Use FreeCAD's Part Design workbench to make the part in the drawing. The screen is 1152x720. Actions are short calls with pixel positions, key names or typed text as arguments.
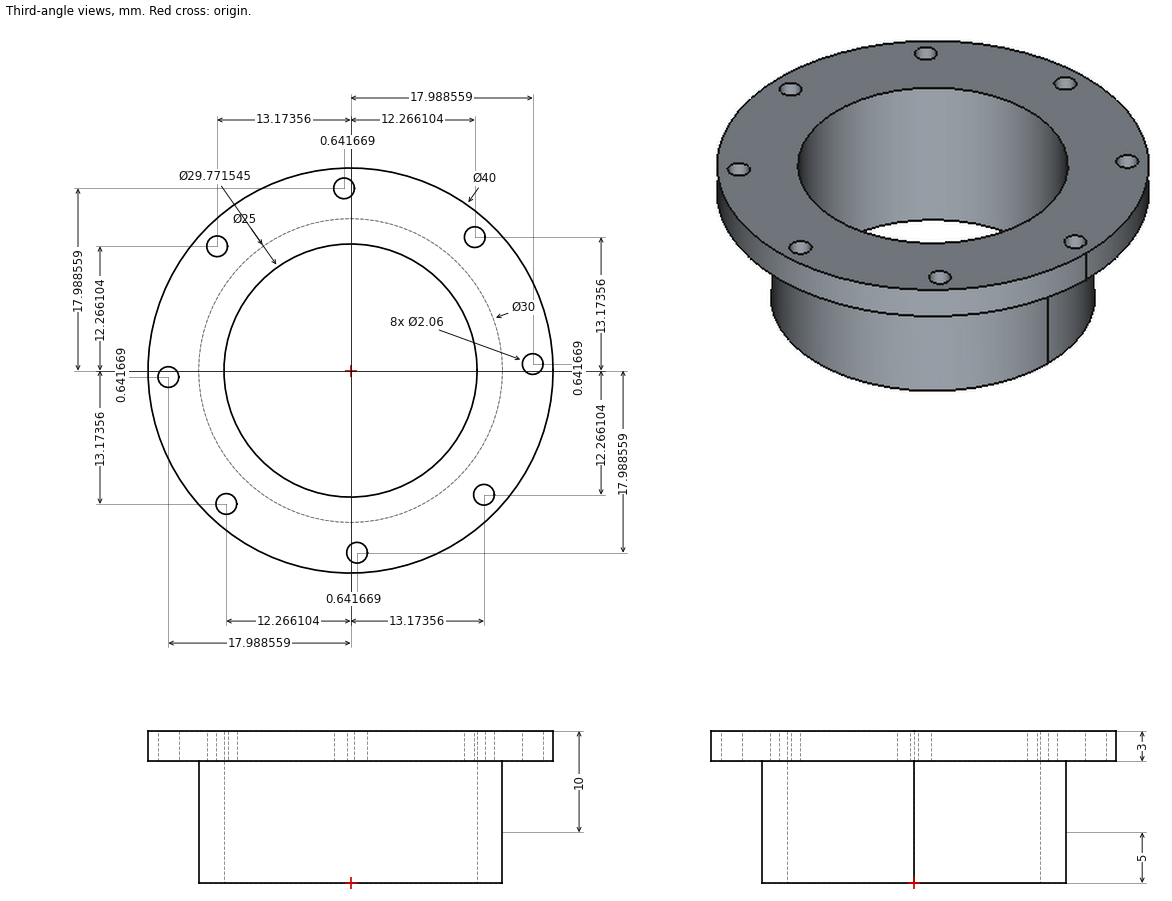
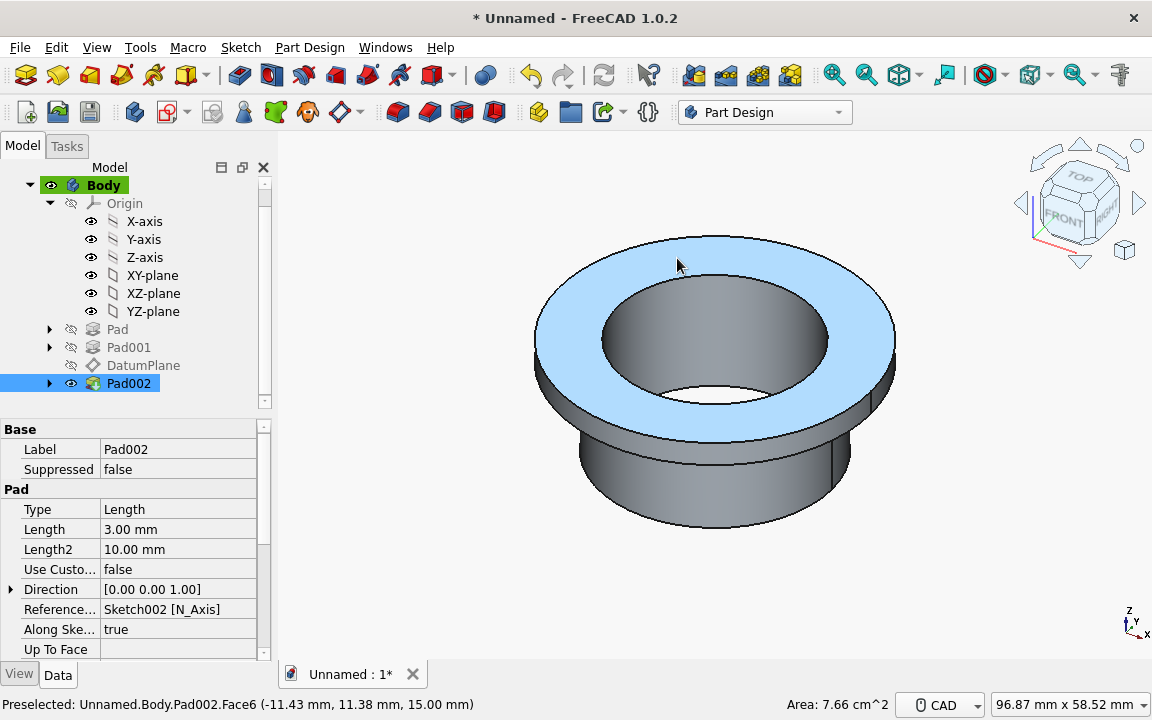
click(168, 112)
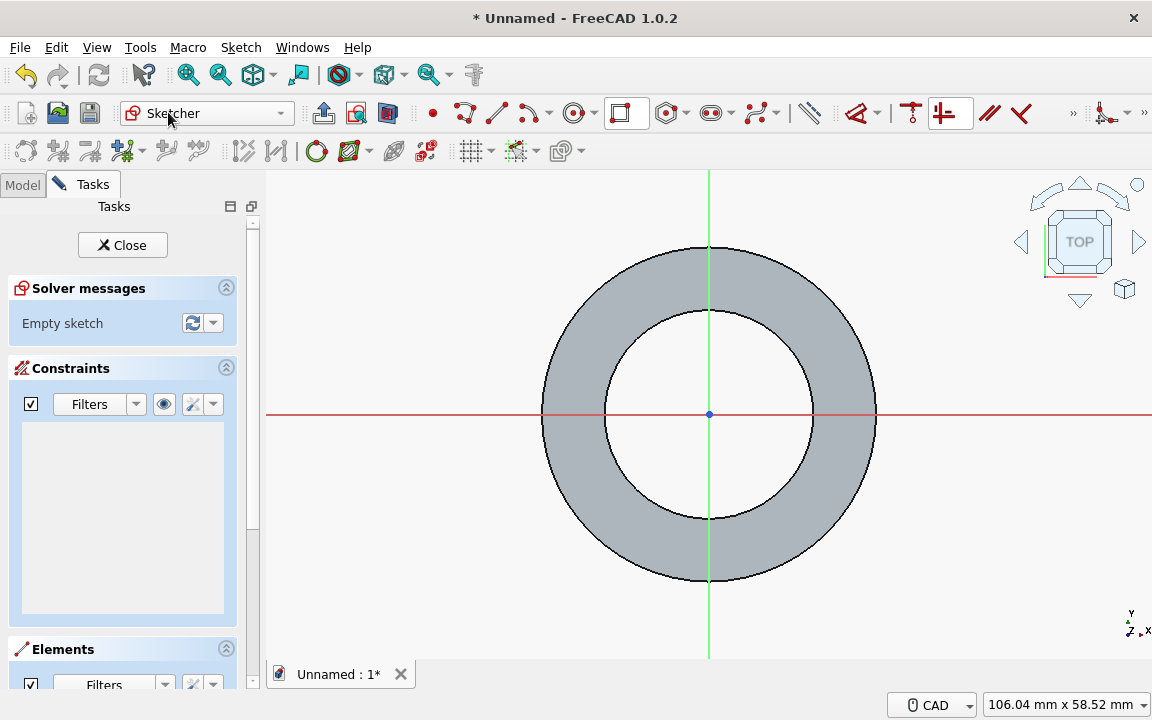
key(g)
key(c)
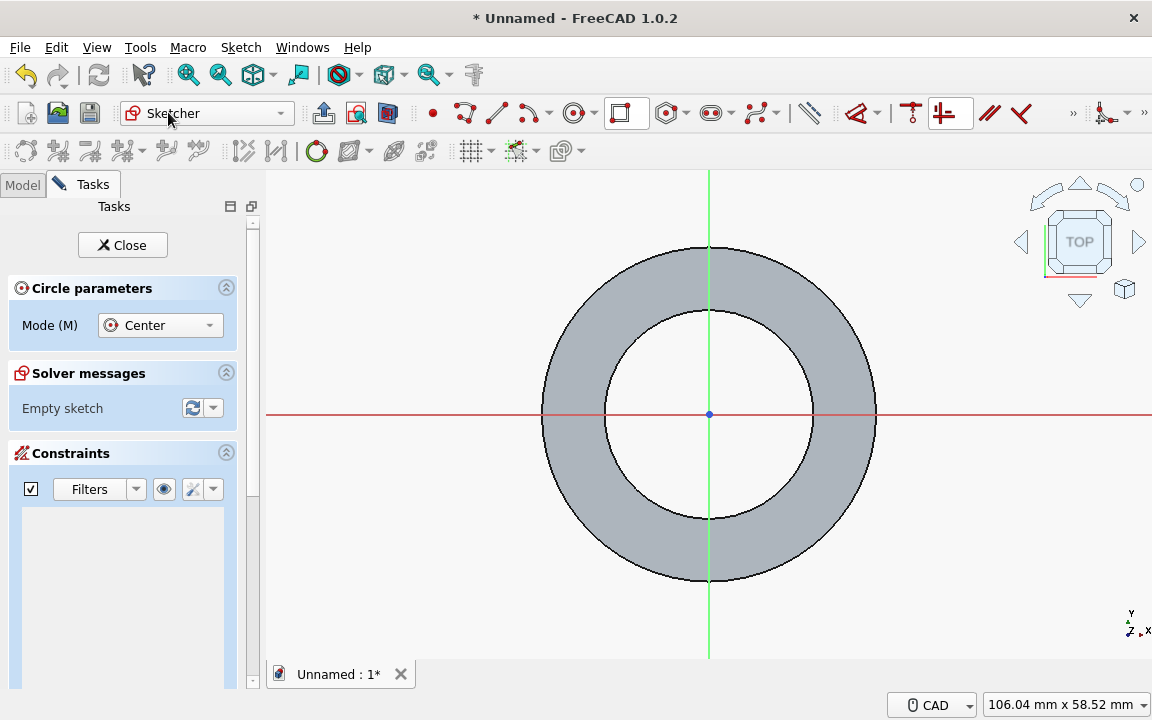
scroll(859, 409, up, 6)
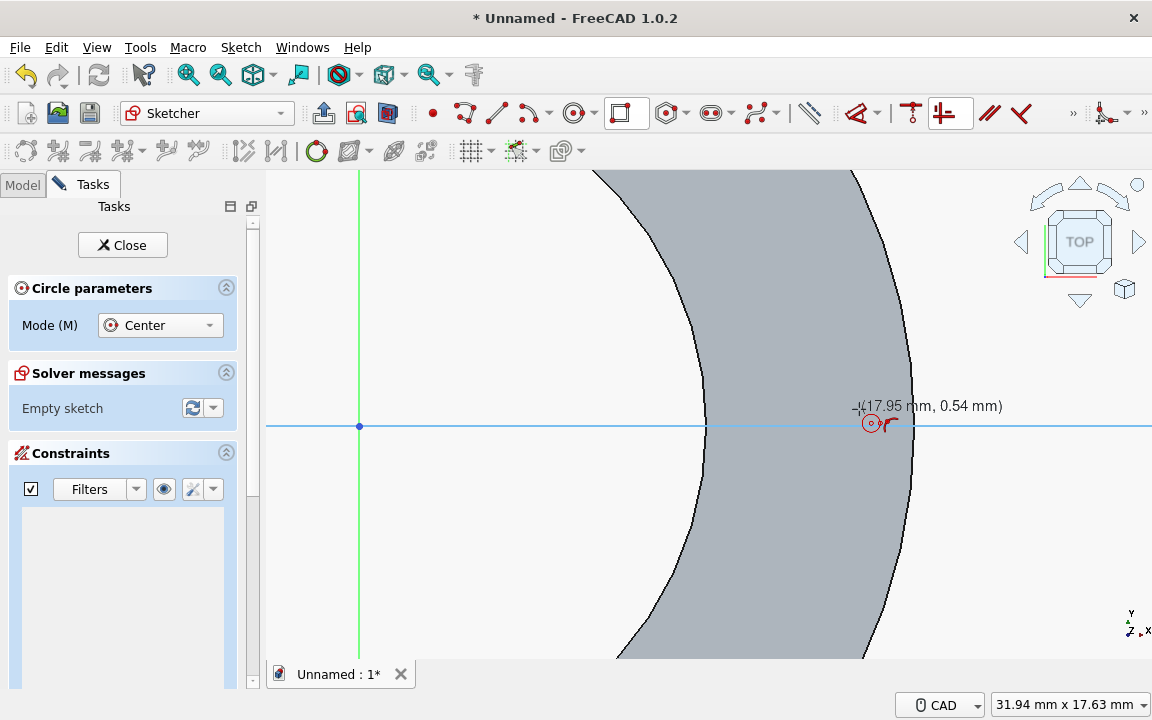
click(858, 408)
click(879, 388)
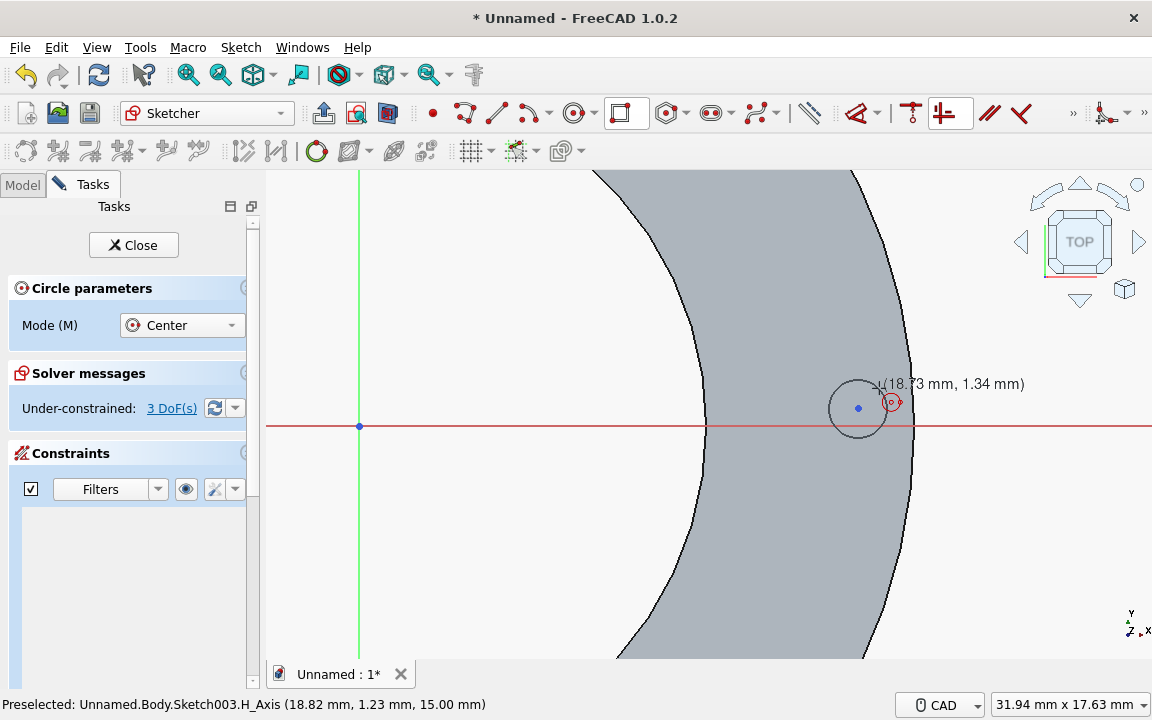
scroll(762, 409, down, 6)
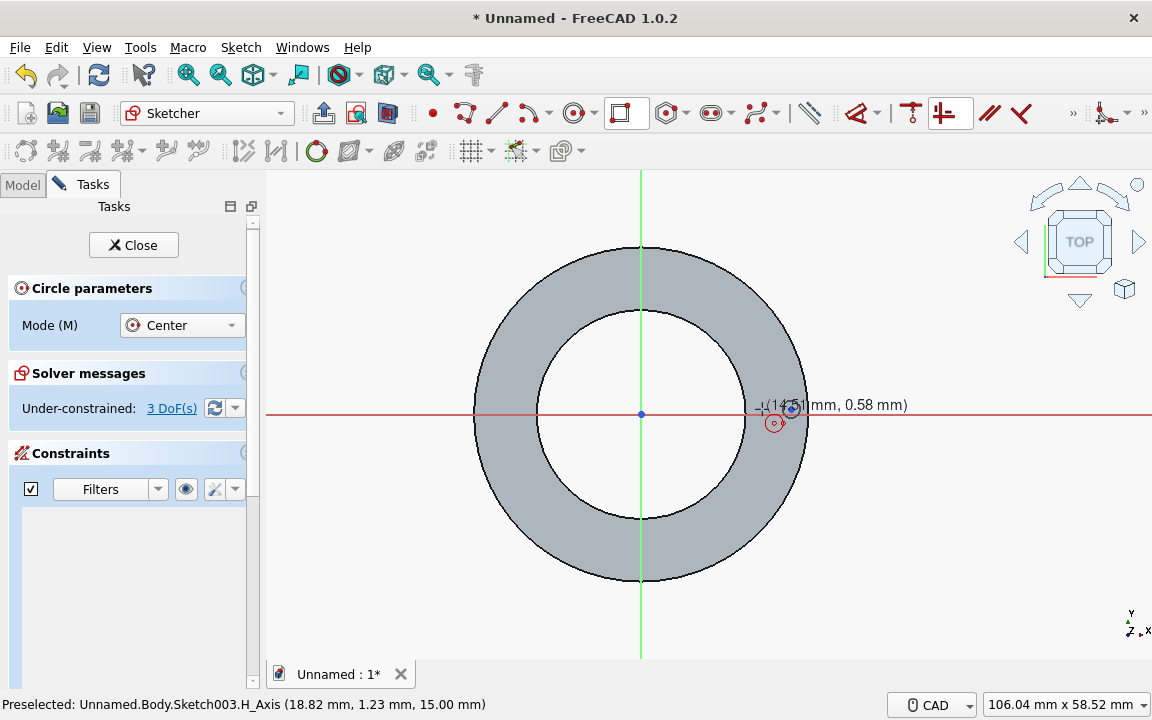
scroll(751, 517, up, 5)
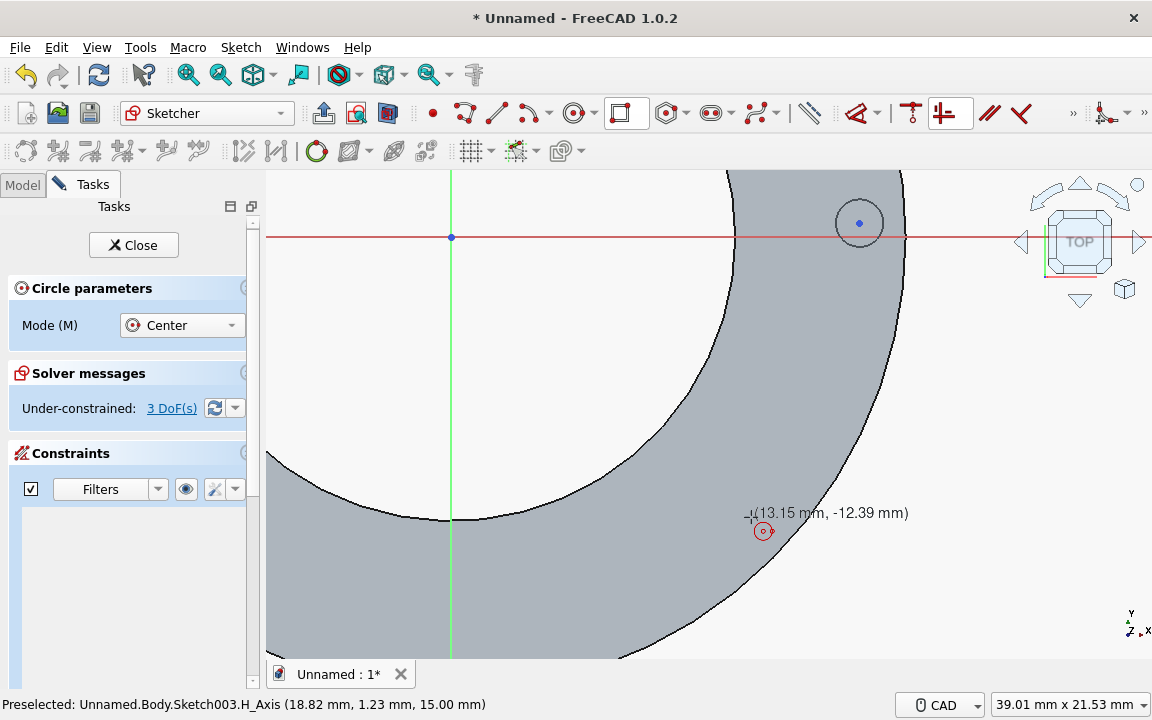
click(751, 516)
click(767, 499)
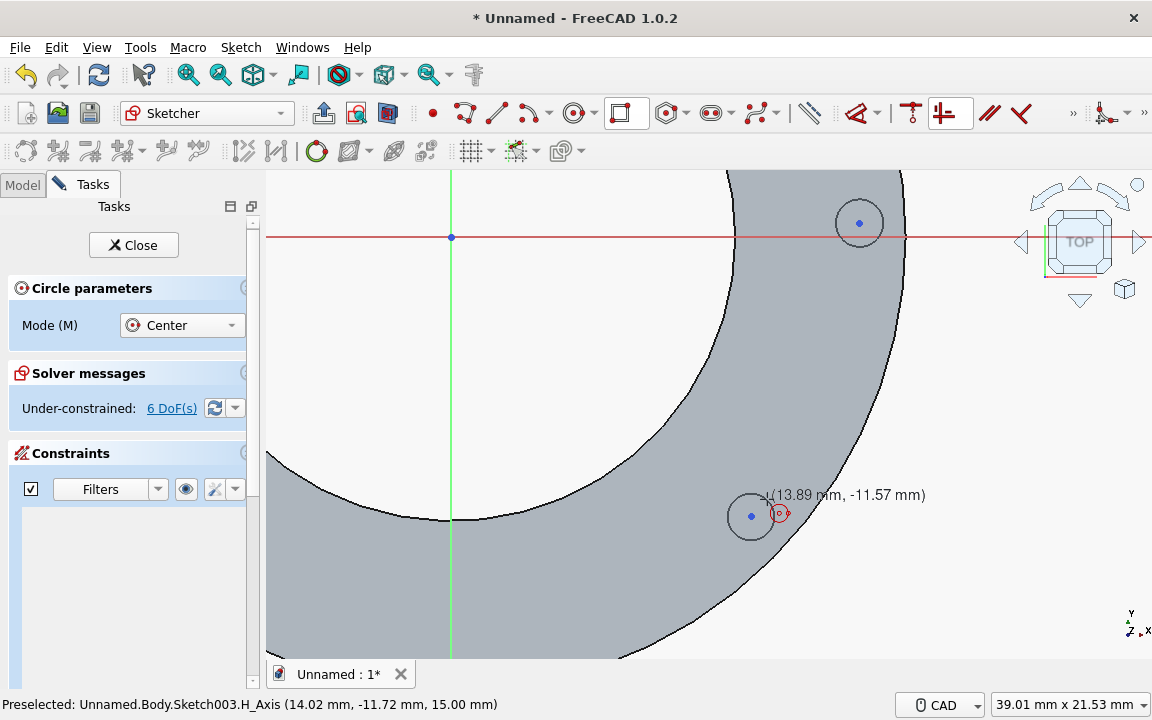
scroll(751, 518, down, 5)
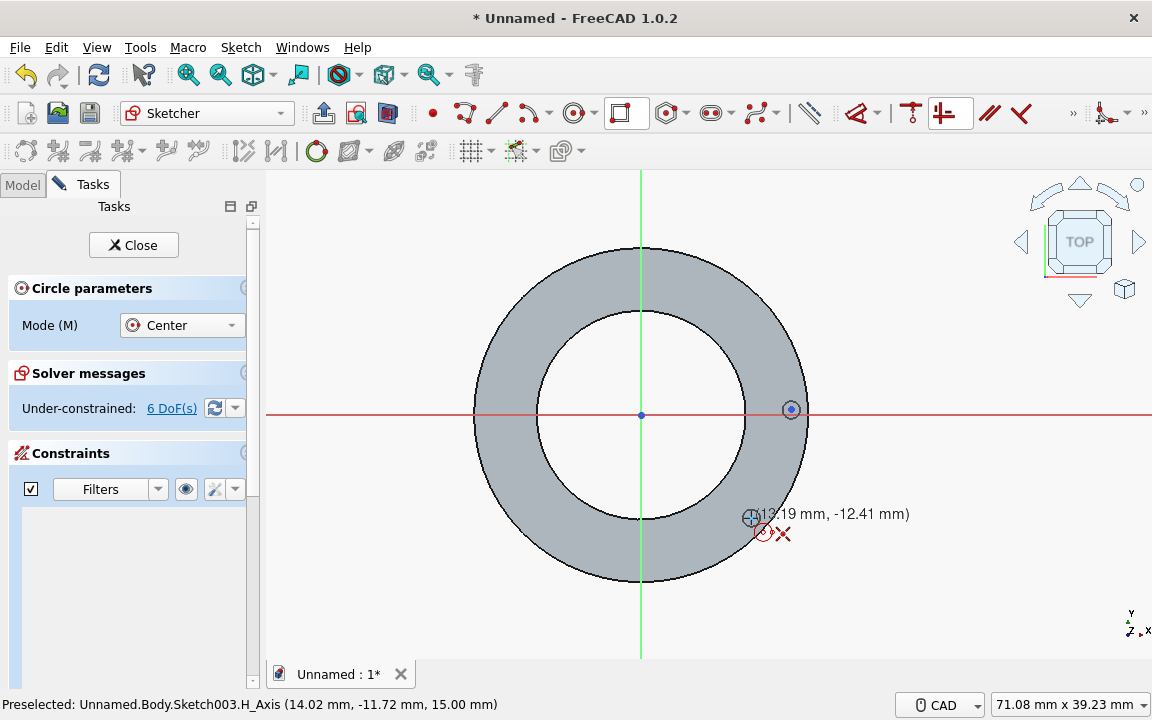
scroll(647, 565, up, 6)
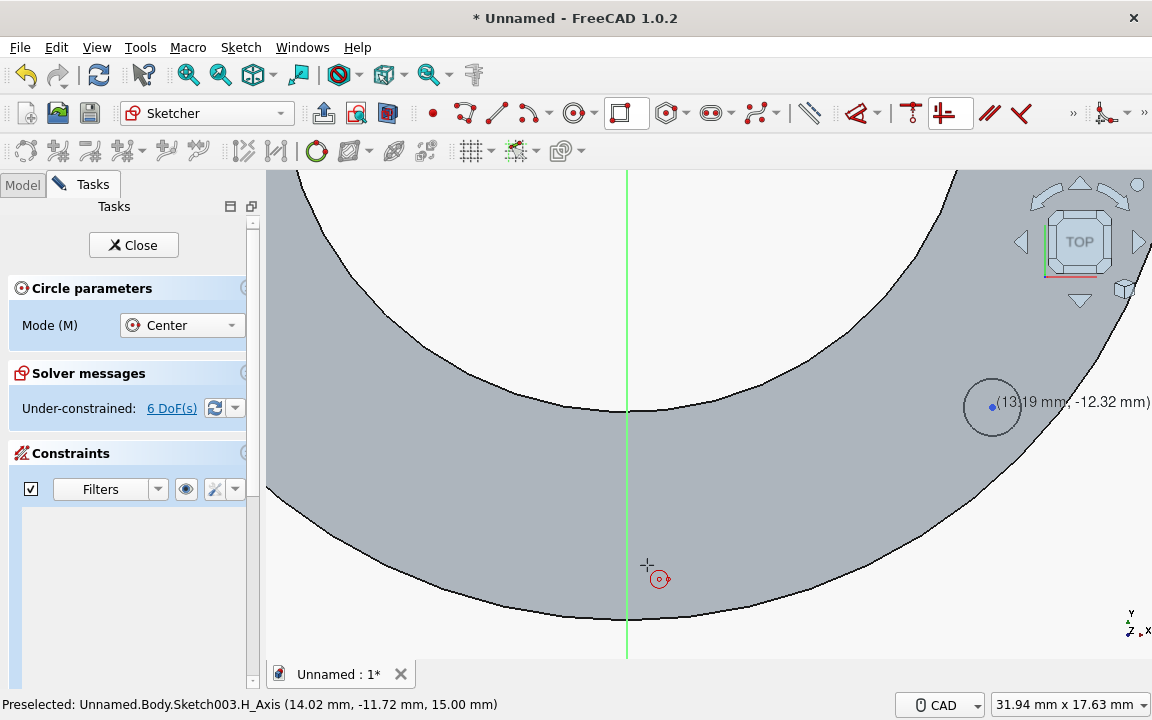
click(644, 565)
click(665, 544)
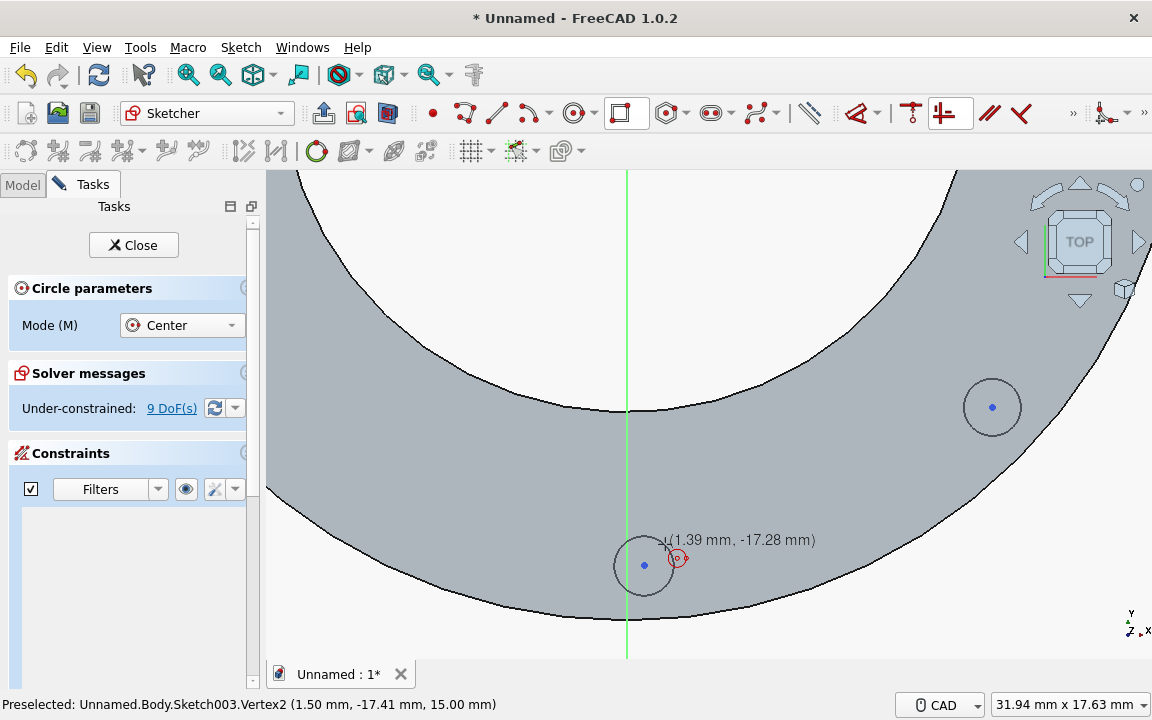
scroll(647, 565, down, 6)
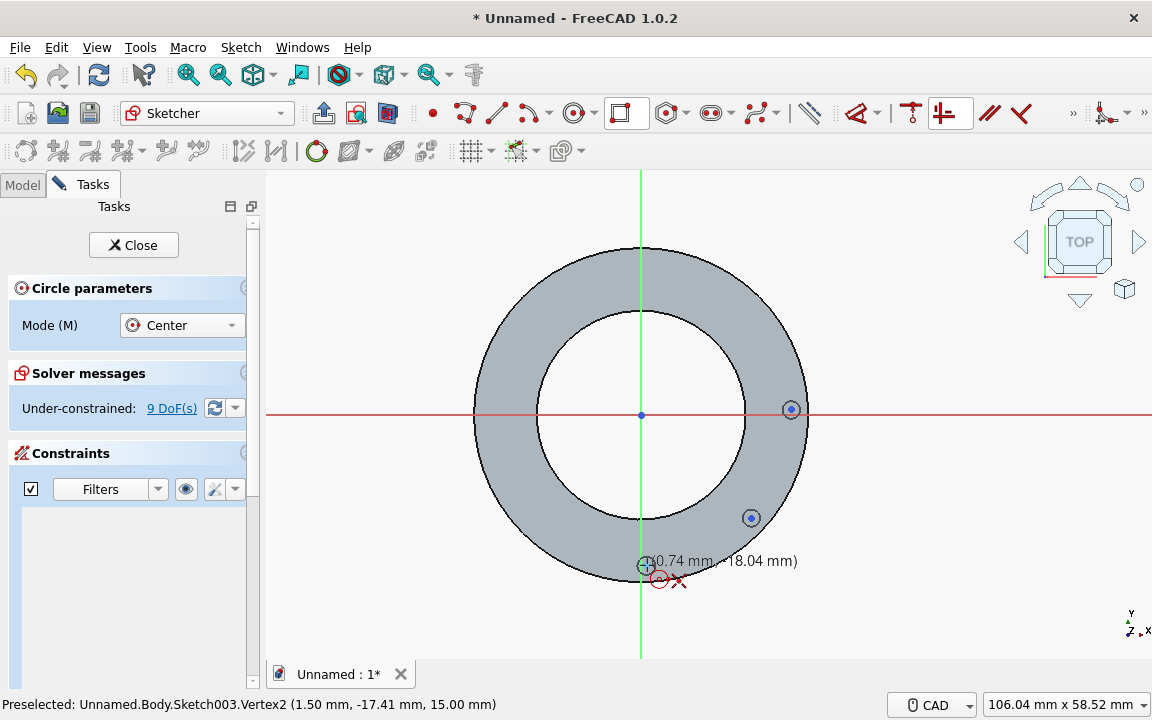
scroll(539, 525, up, 5)